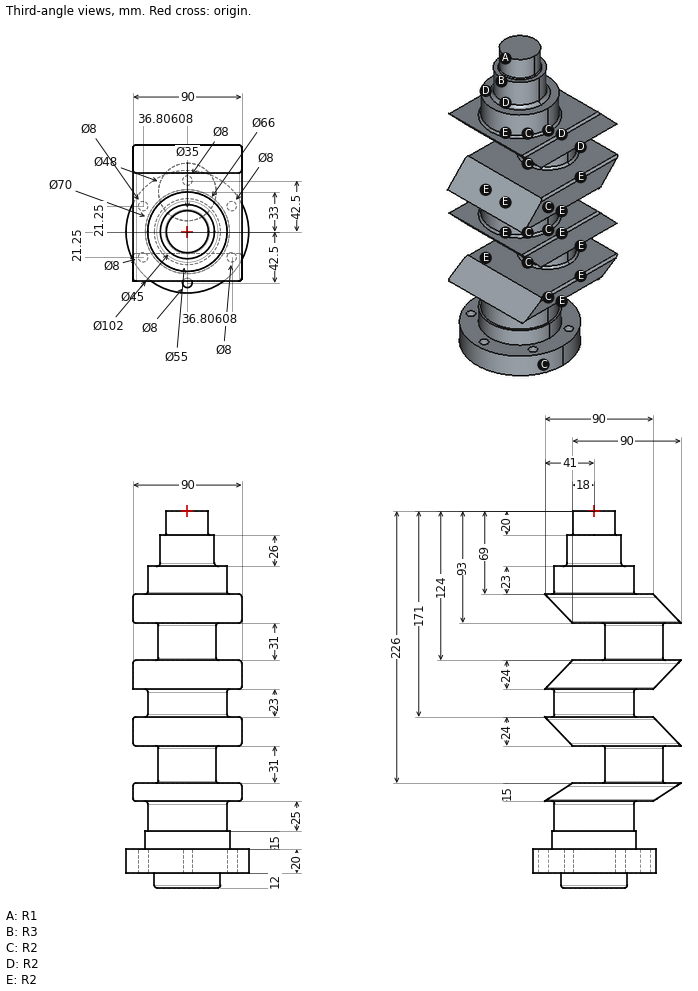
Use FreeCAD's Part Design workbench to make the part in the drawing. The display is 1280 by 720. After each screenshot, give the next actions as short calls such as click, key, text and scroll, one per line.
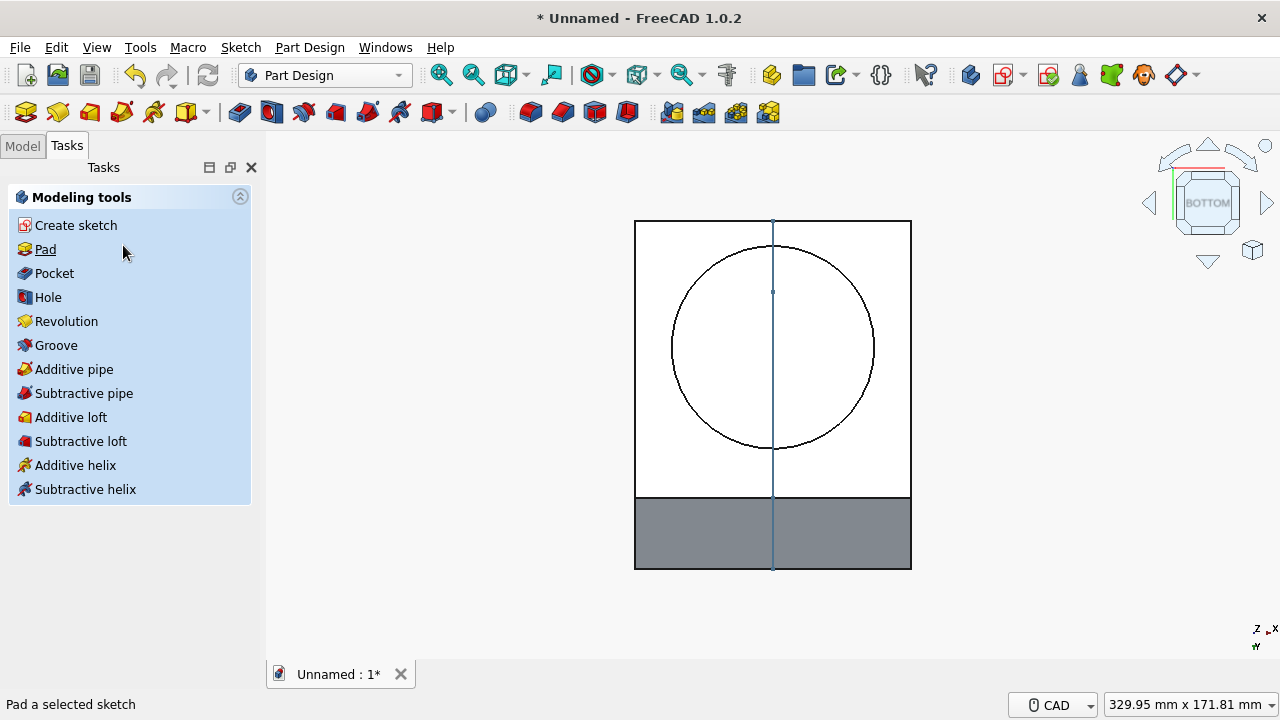
click(26, 112)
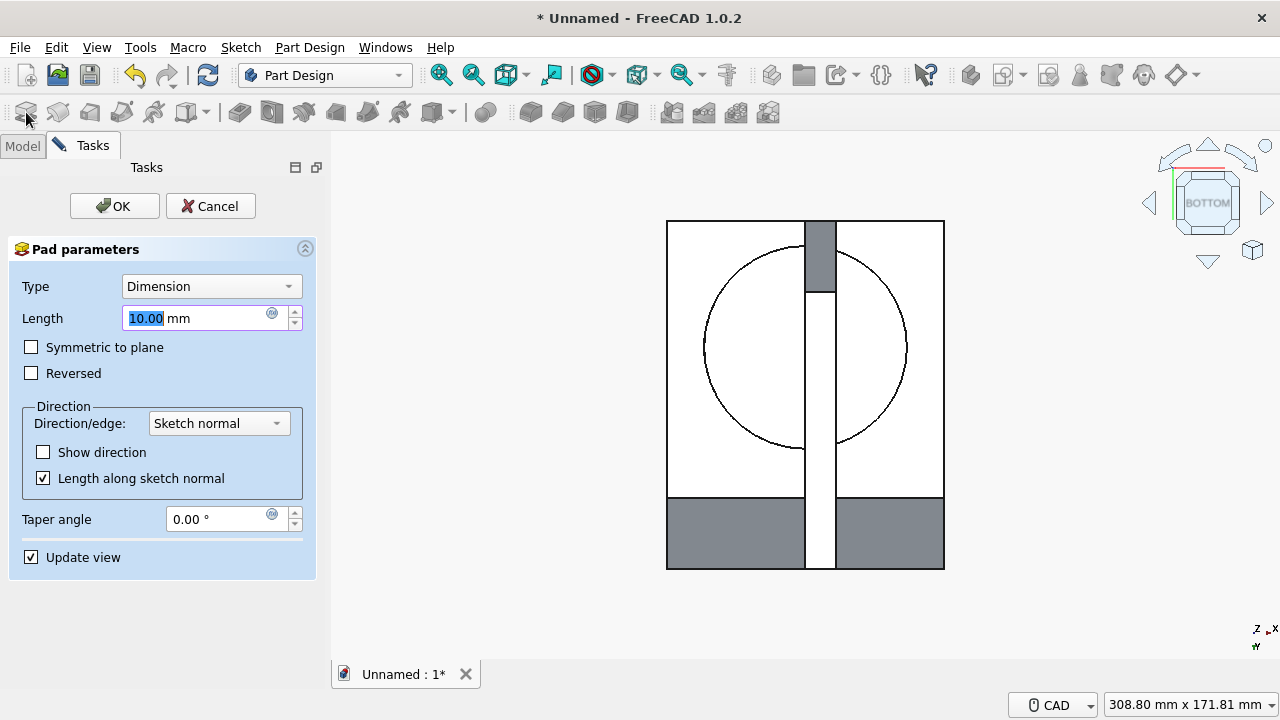
text(90)
key(Tab)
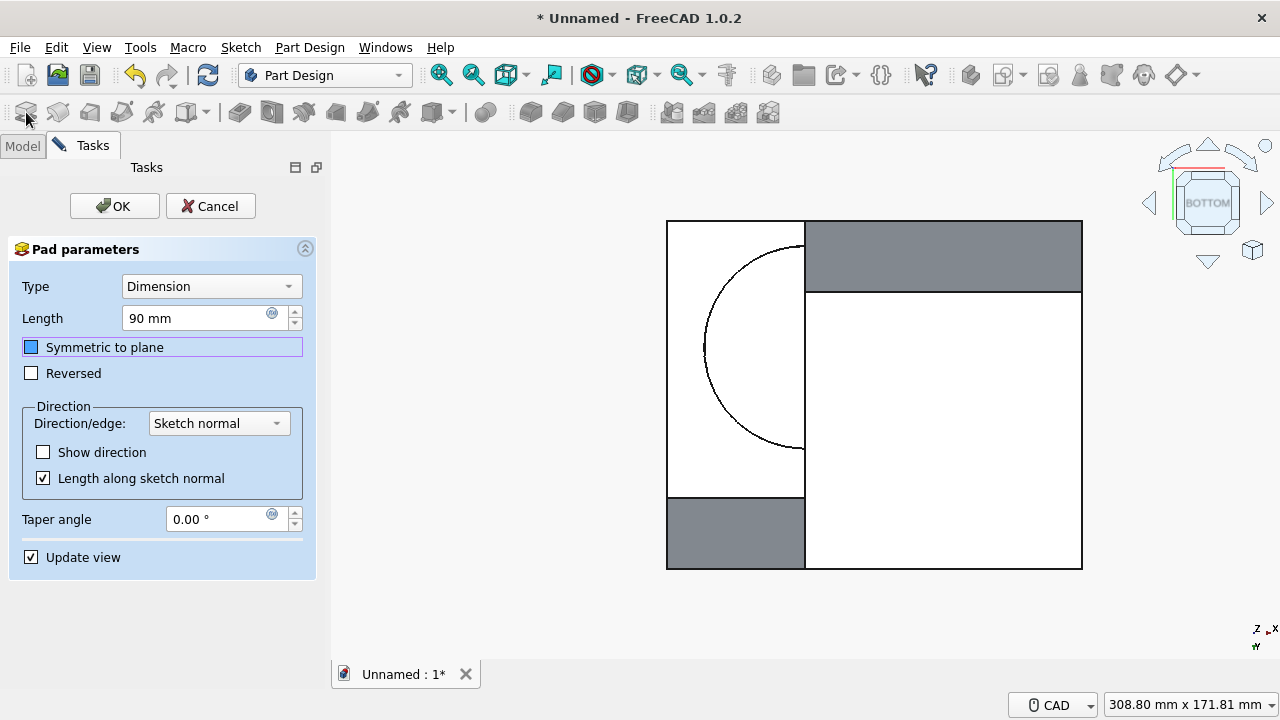
click(30, 347)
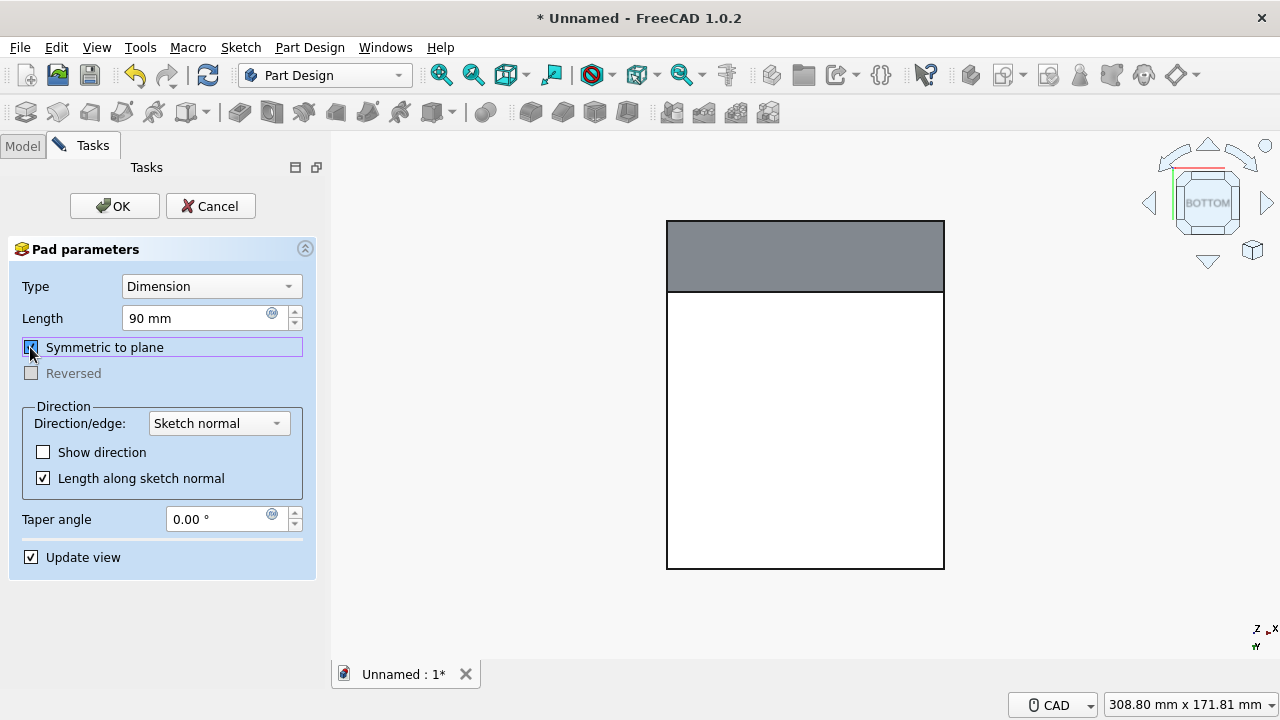
click(115, 206)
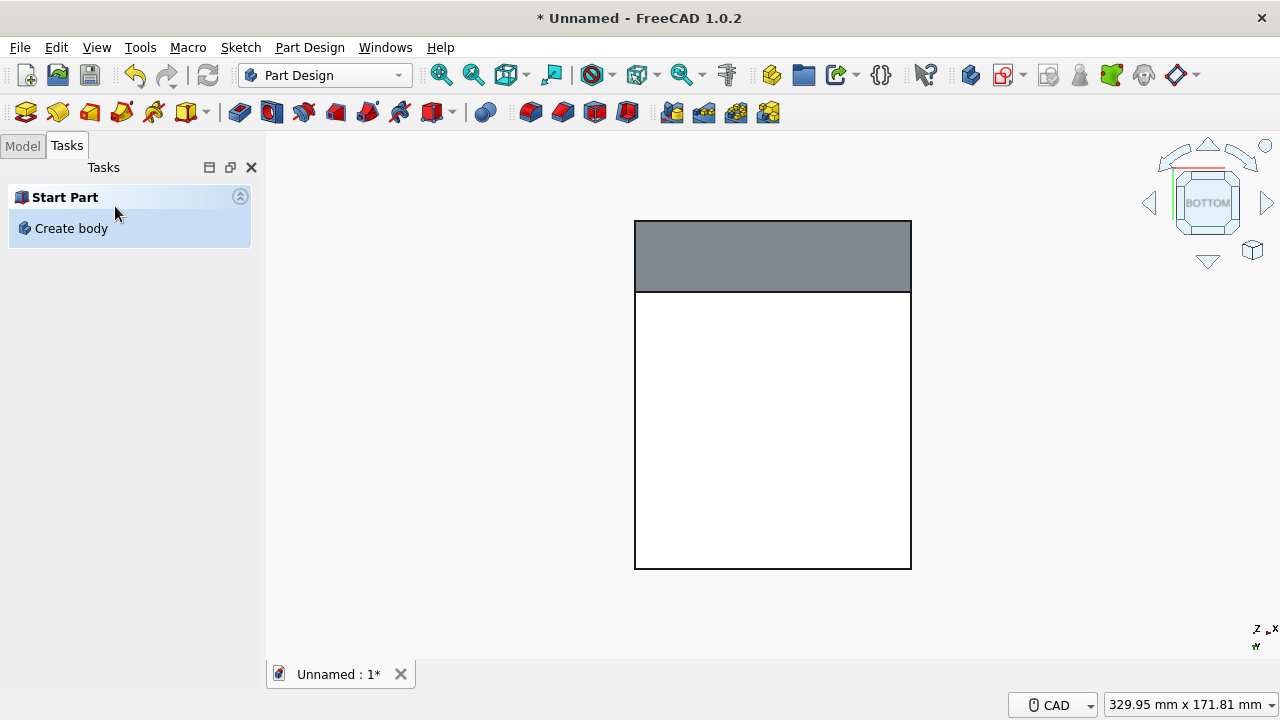
click(773, 429)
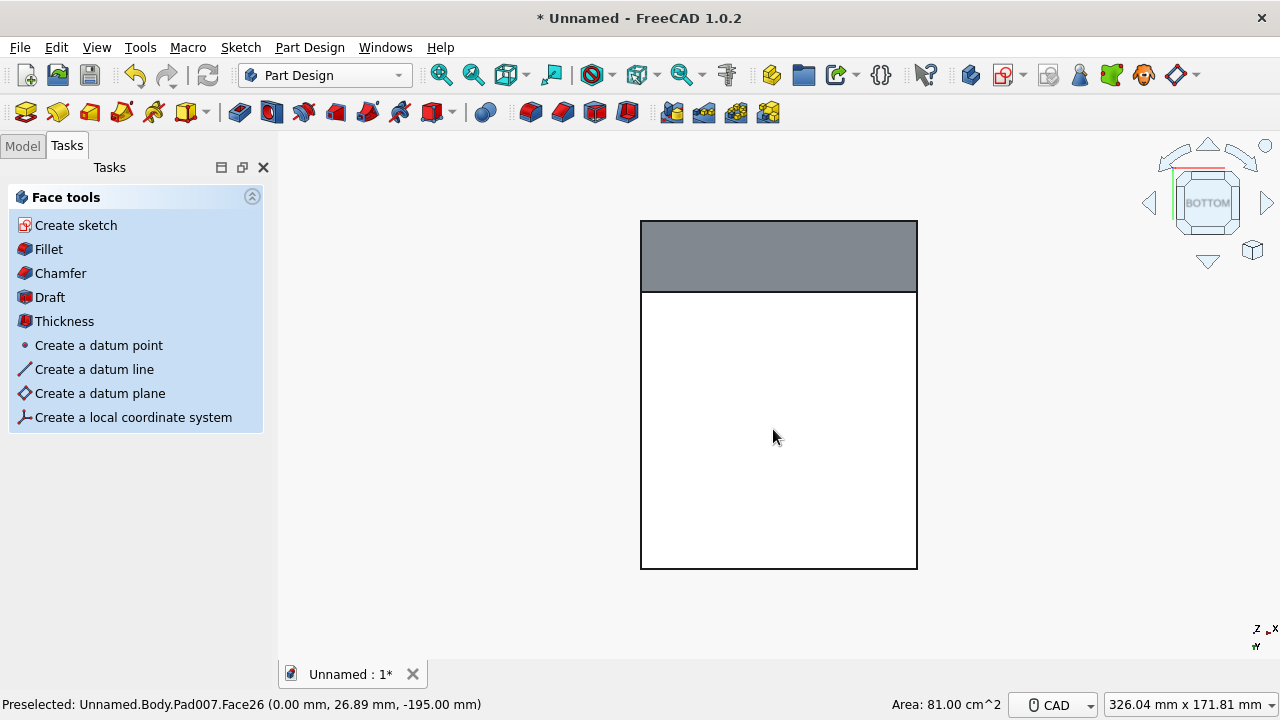
click(1004, 76)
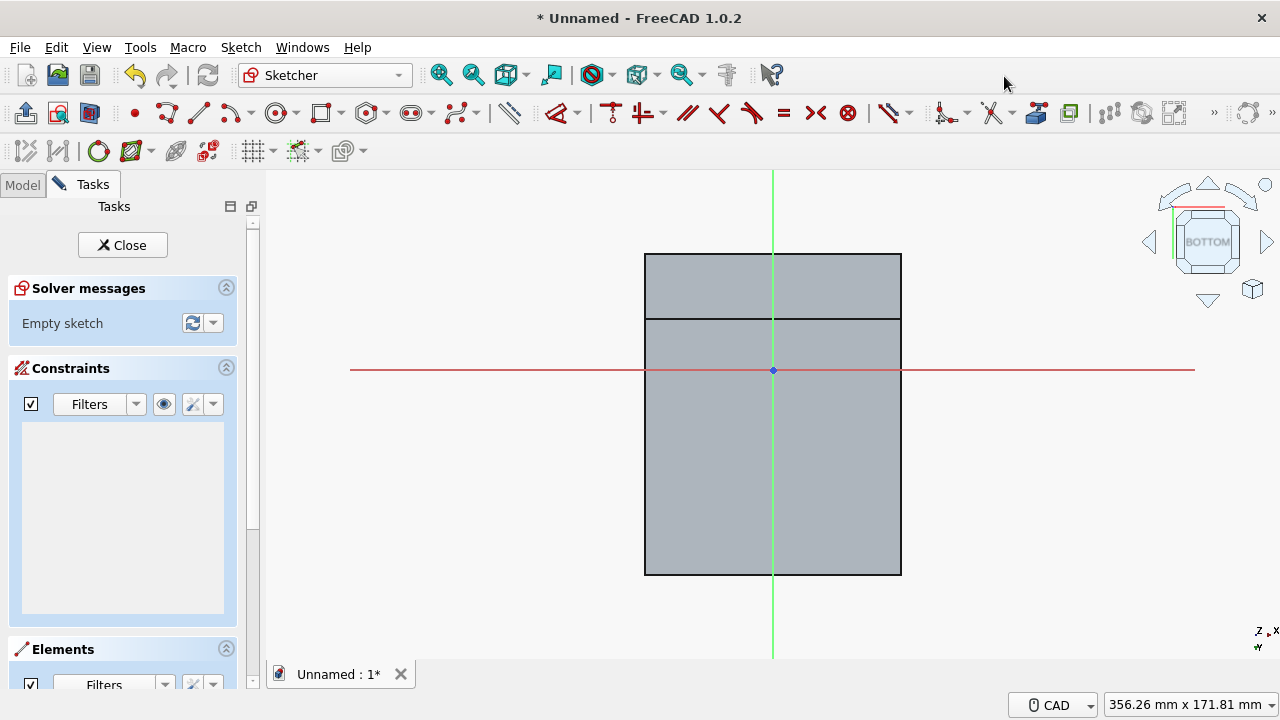
scroll(856, 497, up, 3)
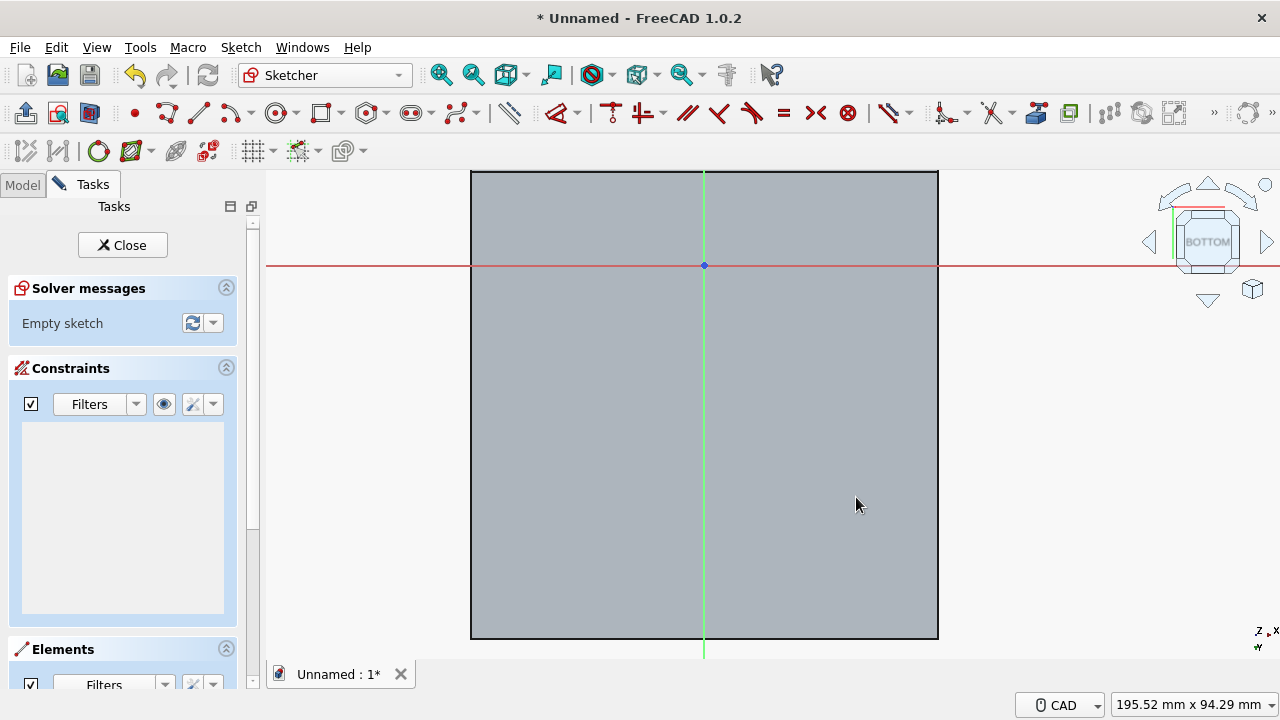
click(276, 114)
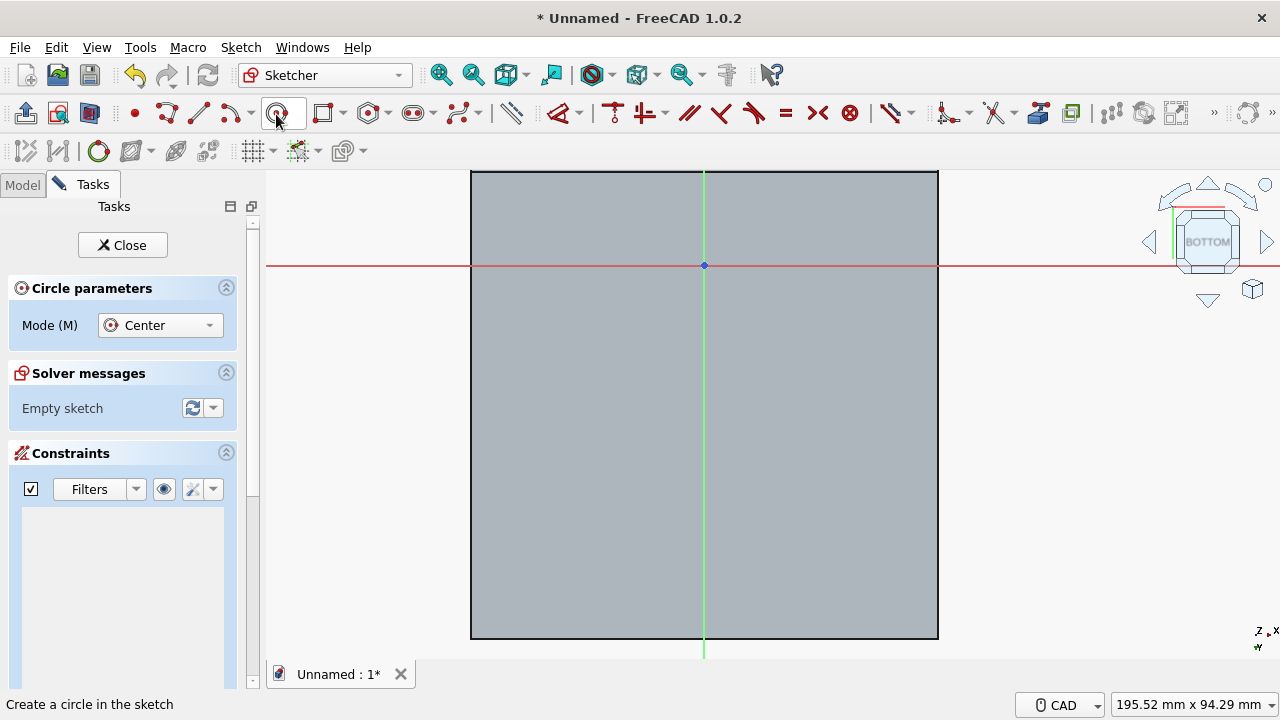
click(704, 437)
move(792, 349)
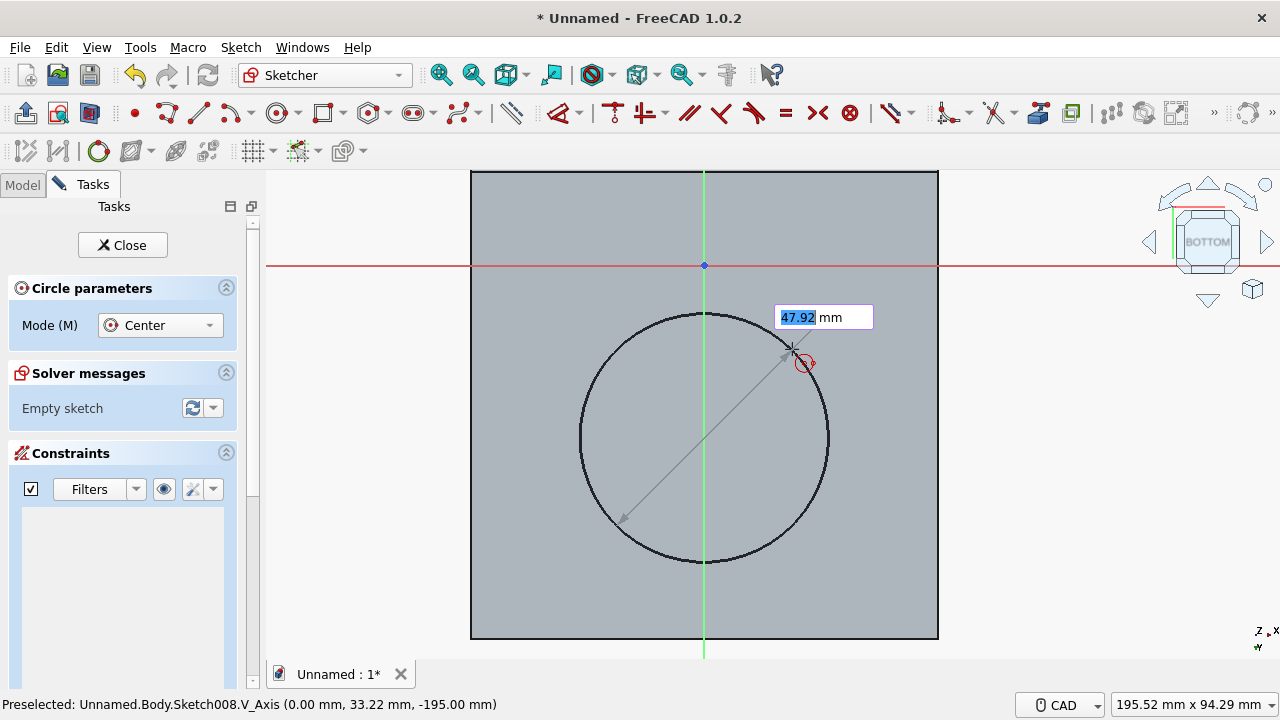
text(48)
key(Return)
key(Escape)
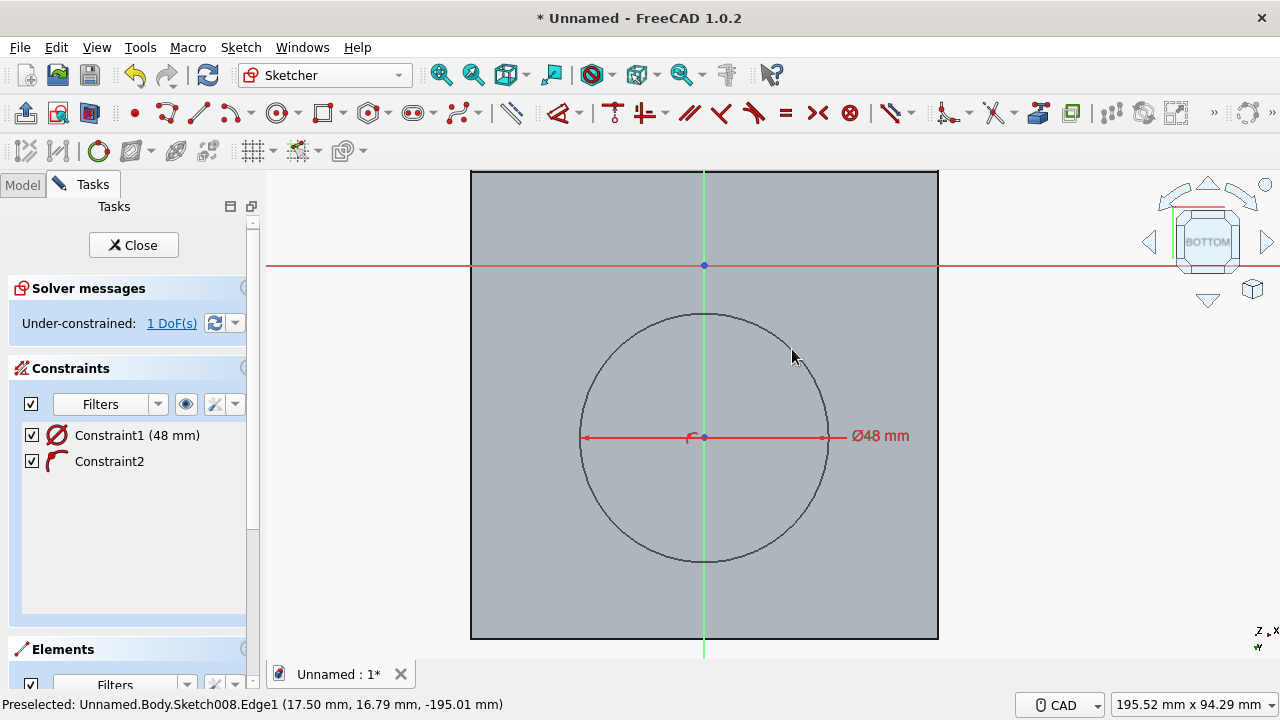
click(558, 114)